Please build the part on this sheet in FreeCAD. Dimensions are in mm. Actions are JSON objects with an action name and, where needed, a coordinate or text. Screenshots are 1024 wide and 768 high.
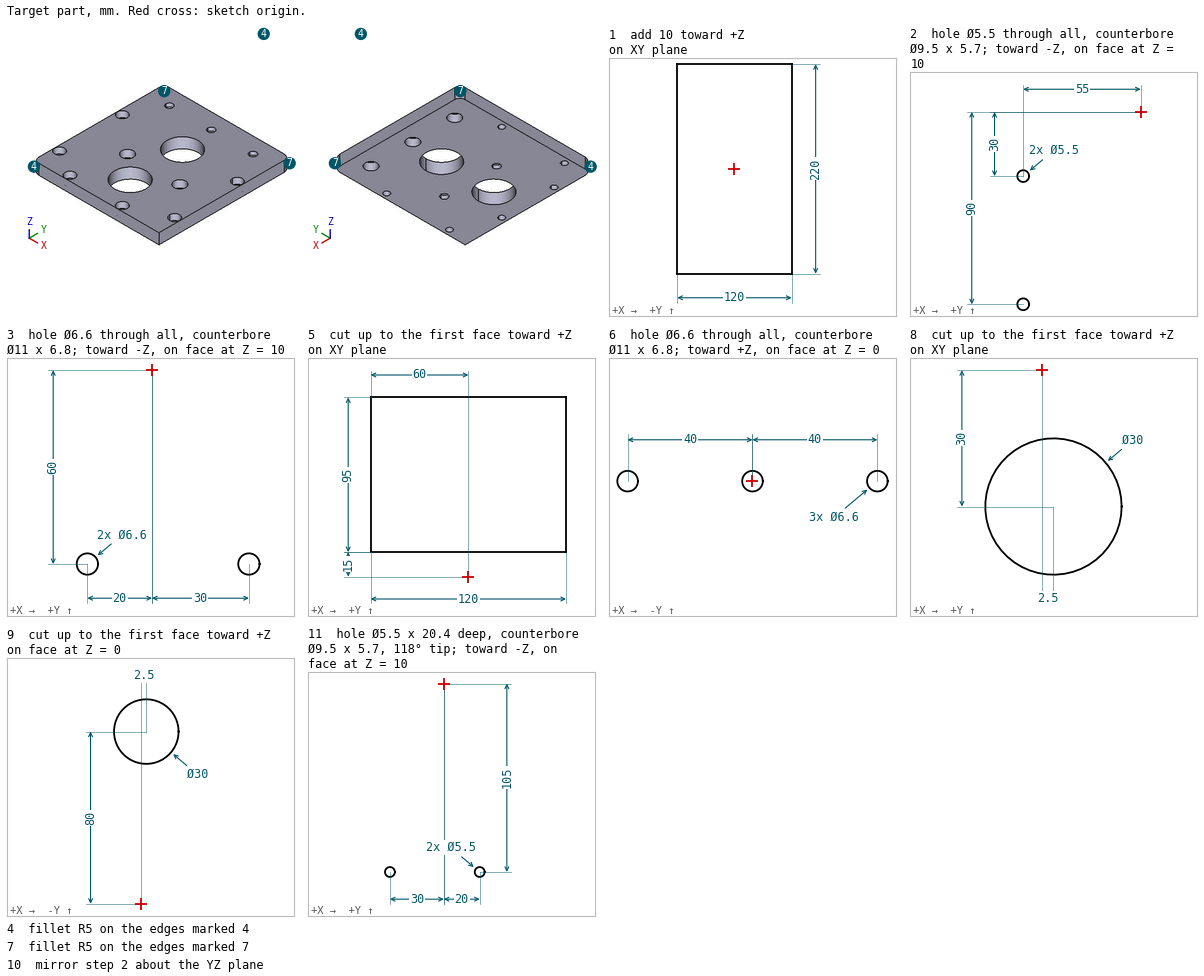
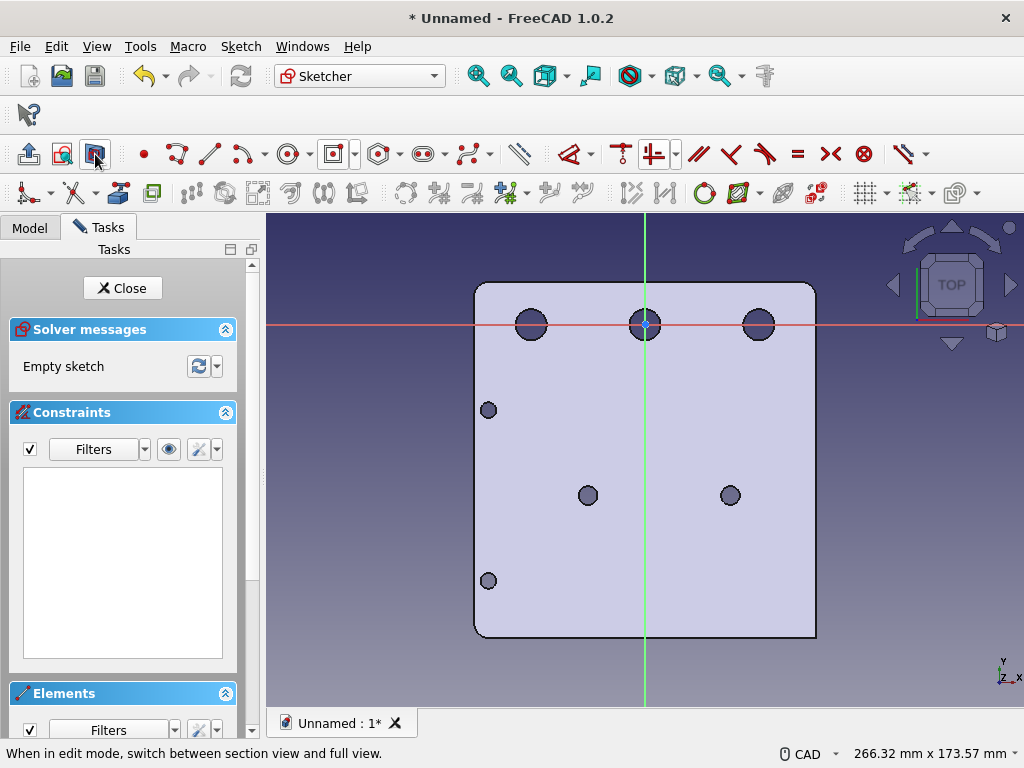
{"action": "scroll", "coordinate": [714, 331], "scroll_direction": "up", "scroll_amount": 4}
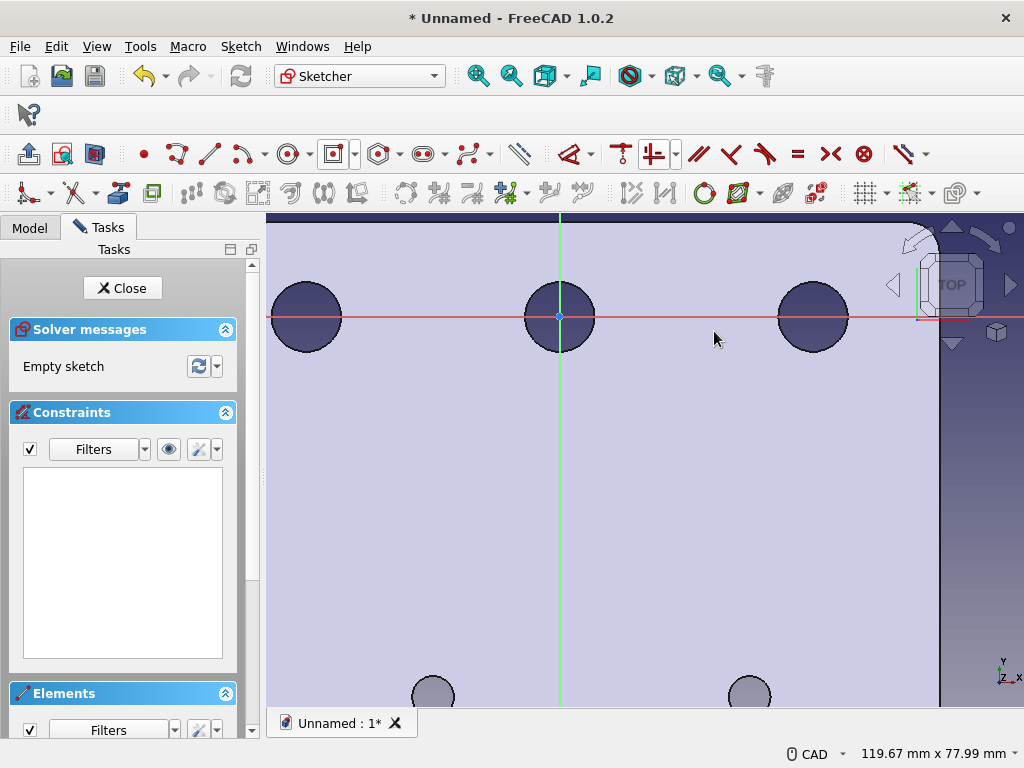
{"action": "left_click", "coordinate": [288, 154]}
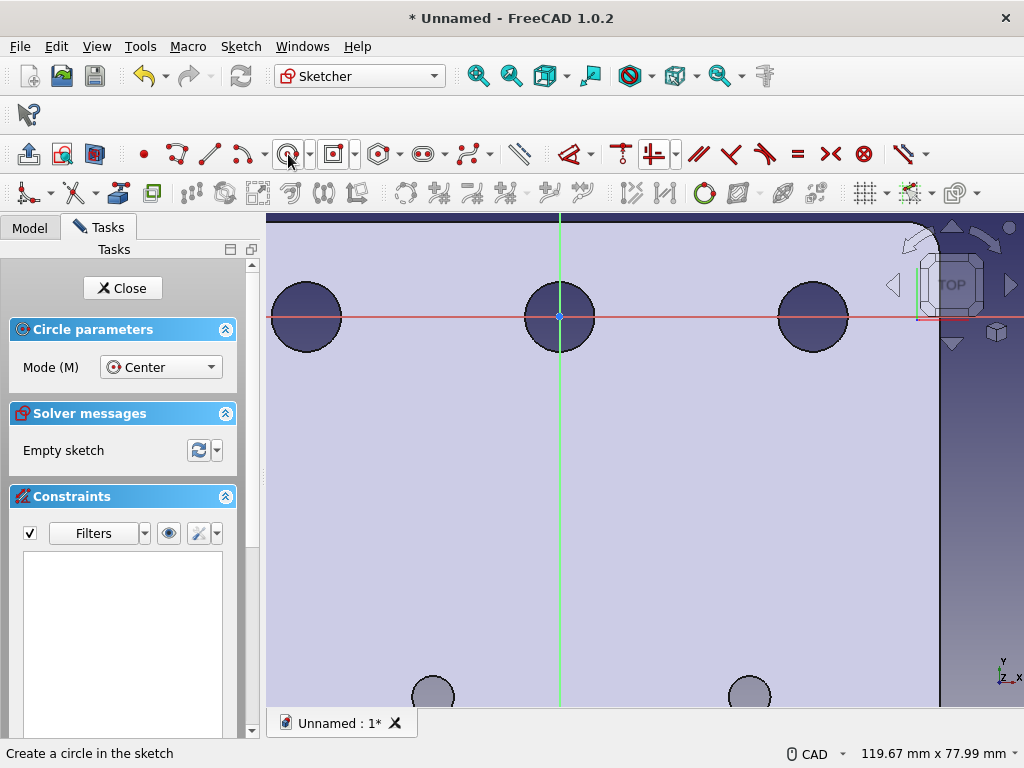
{"action": "left_click", "coordinate": [576, 507]}
{"action": "left_click", "coordinate": [643, 440]}
{"action": "key", "text": "Escape"}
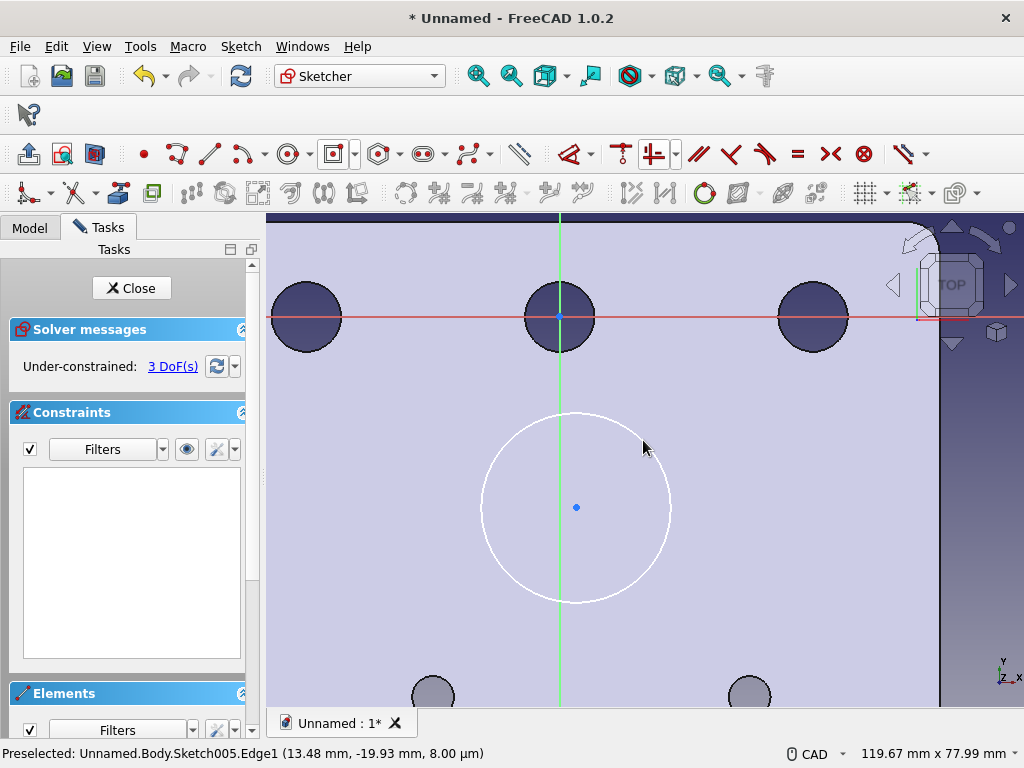
{"action": "left_click", "coordinate": [568, 154]}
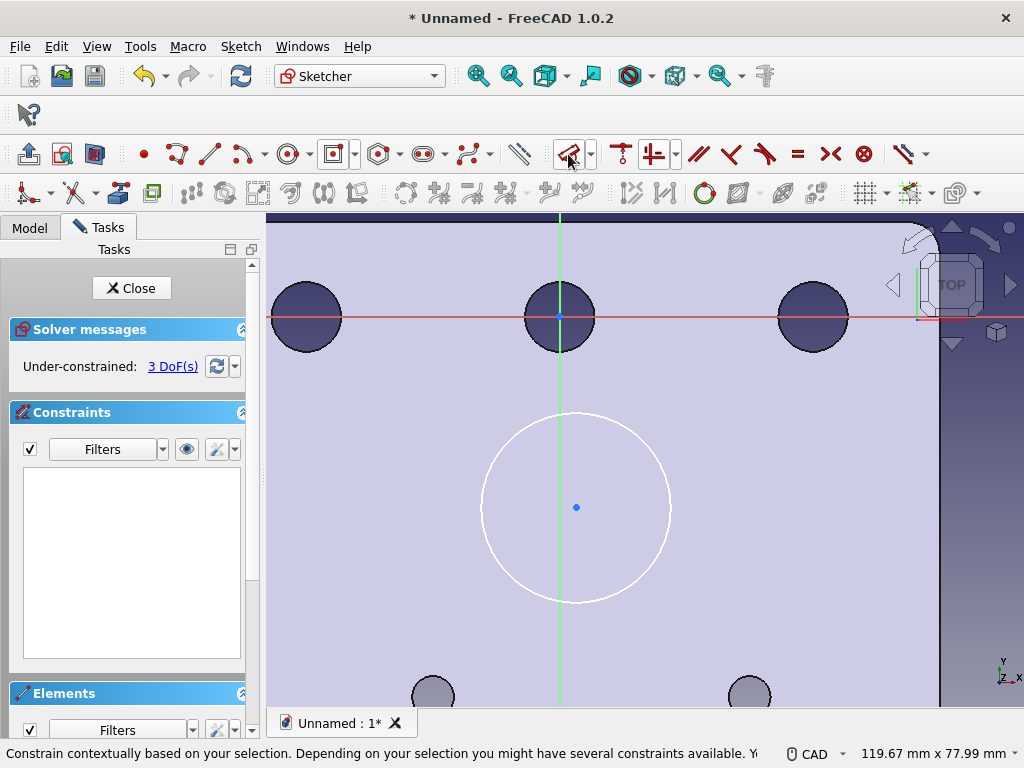
{"action": "left_click", "coordinate": [643, 441]}
{"action": "left_click", "coordinate": [666, 418]}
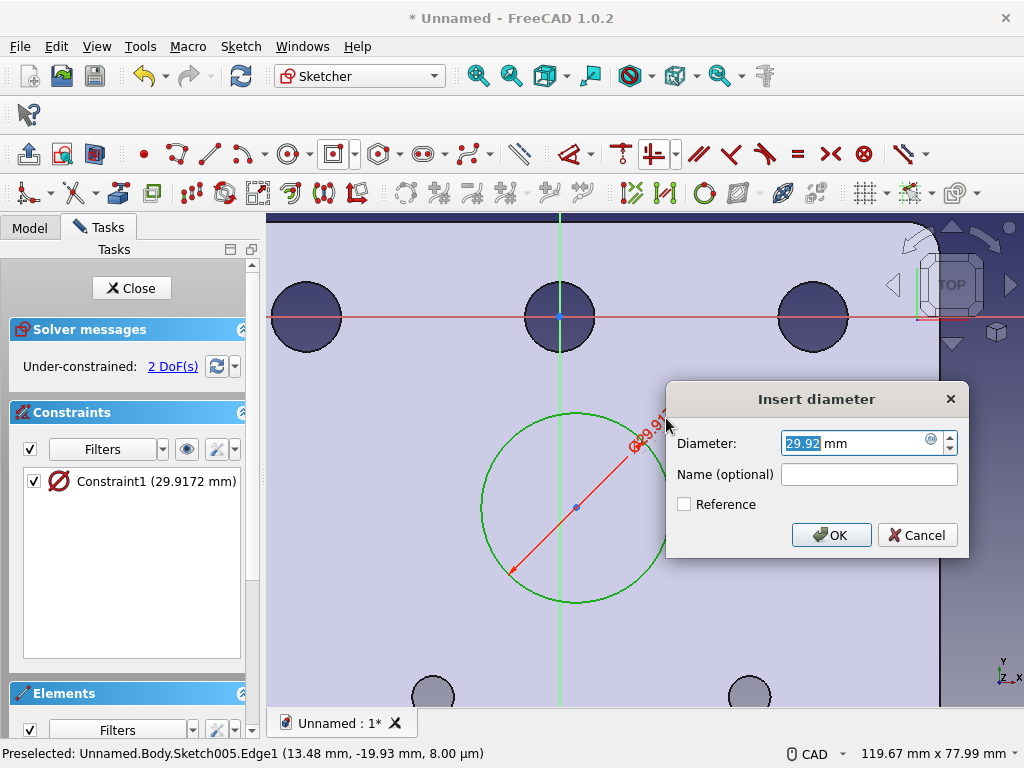
{"action": "type", "text": "30"}
{"action": "key", "text": "Return"}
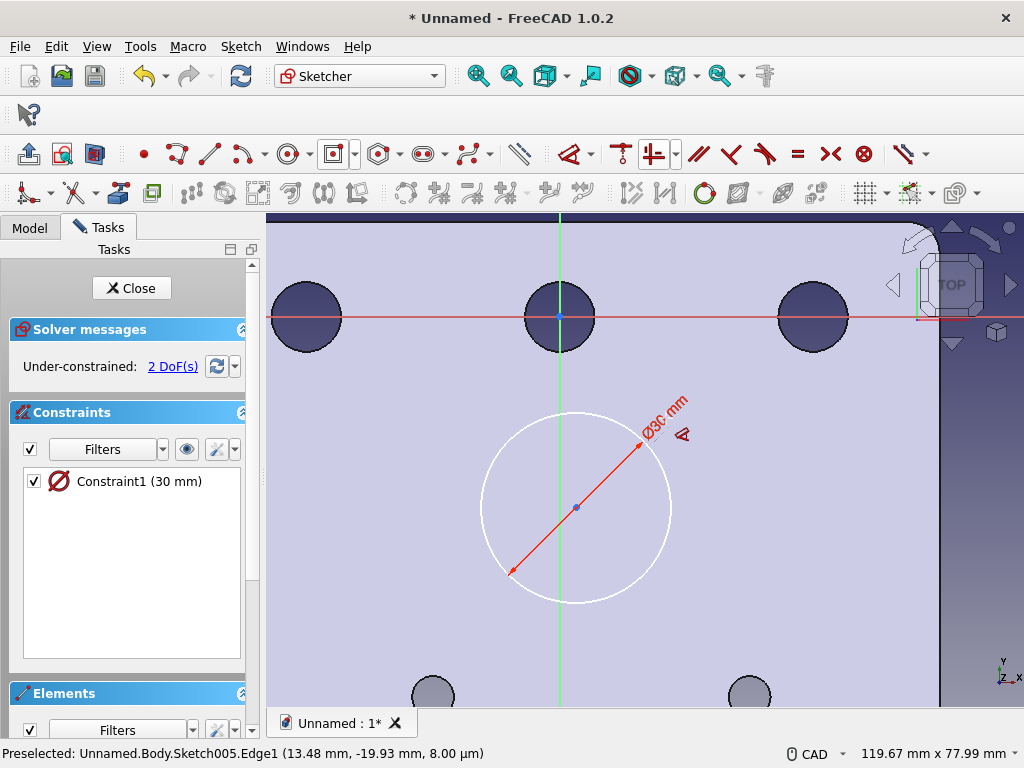
{"action": "left_click", "coordinate": [576, 508]}
{"action": "left_click", "coordinate": [526, 369]}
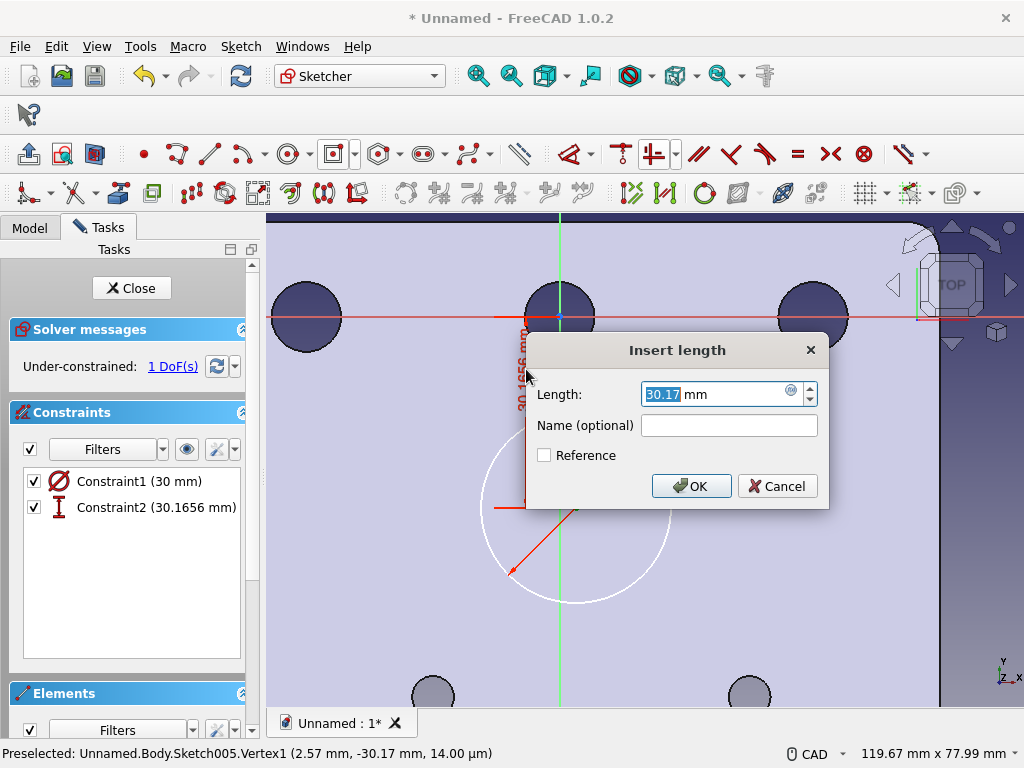
{"action": "type", "text": "30"}
{"action": "key", "text": "Return"}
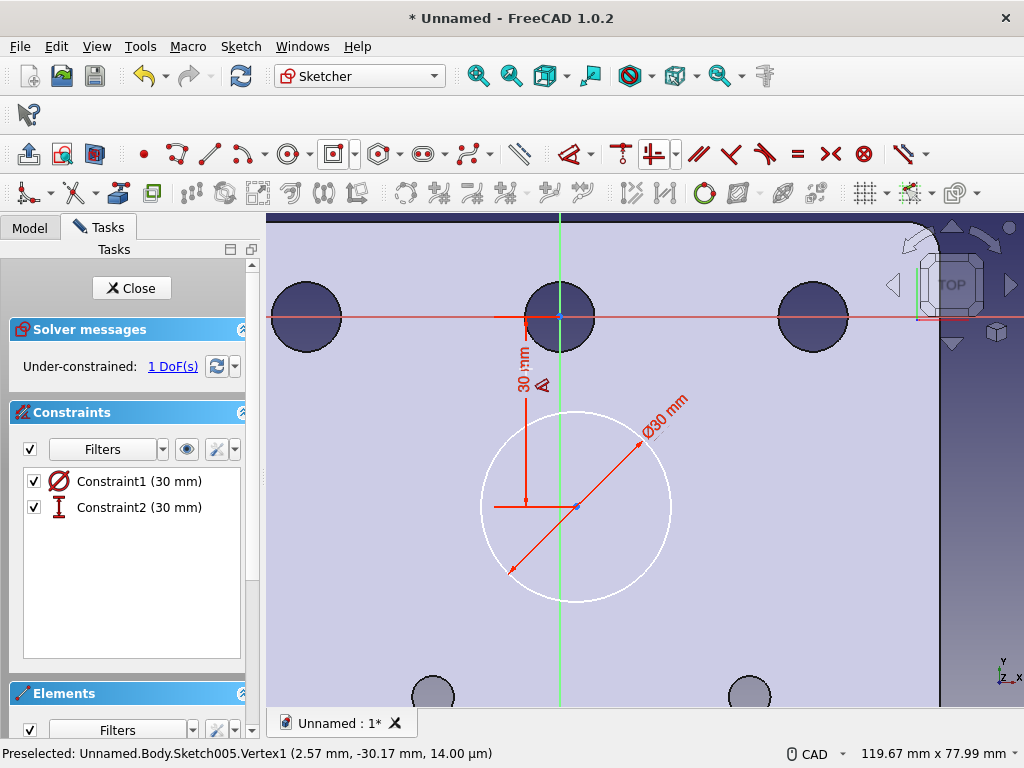
{"action": "scroll", "coordinate": [576, 507], "scroll_direction": "up", "scroll_amount": 5}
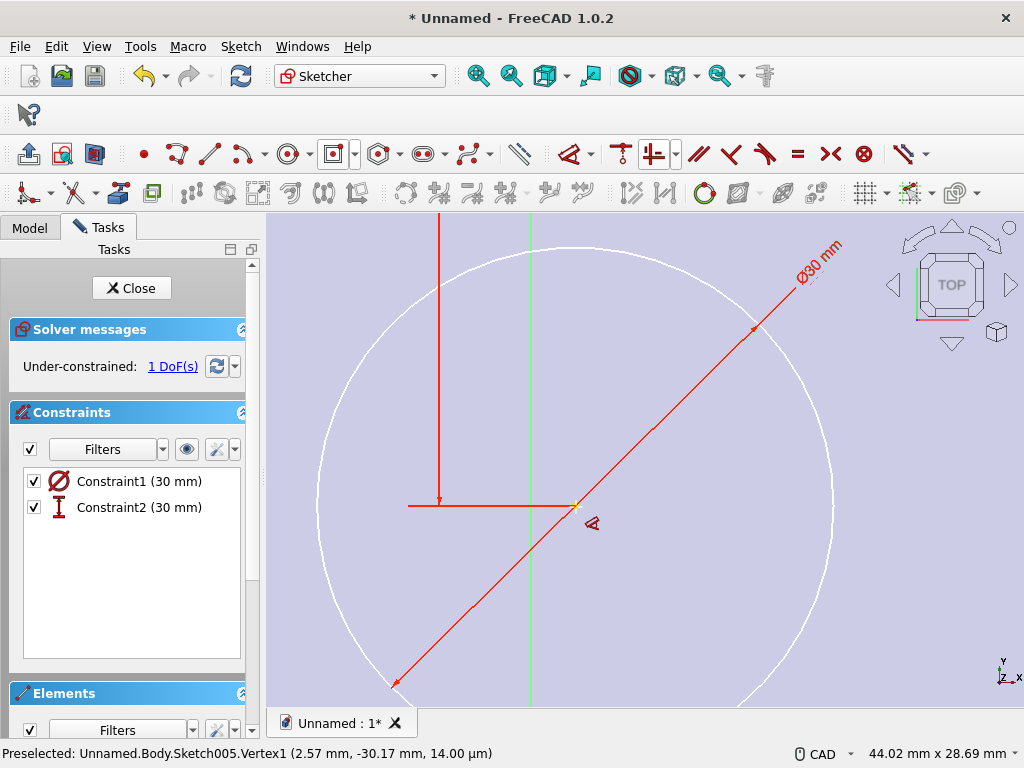
{"action": "left_click", "coordinate": [575, 506]}
{"action": "left_click", "coordinate": [553, 540]}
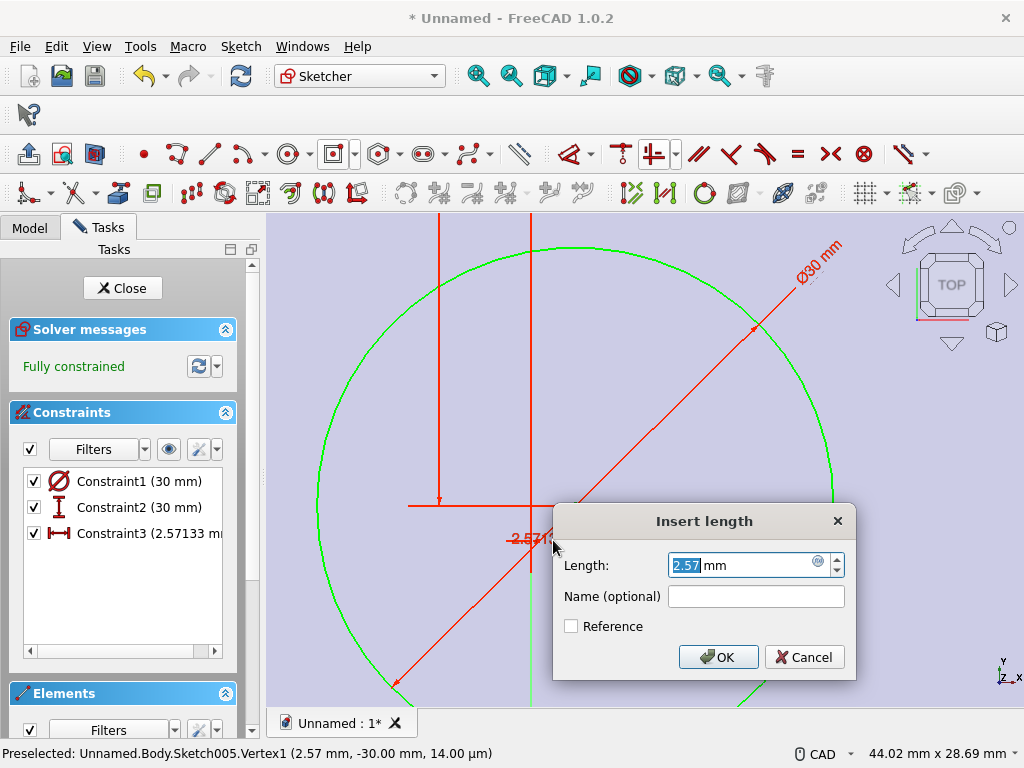
{"action": "type", "text": "2.5"}
{"action": "key", "text": "Return"}
{"action": "key", "text": "Escape"}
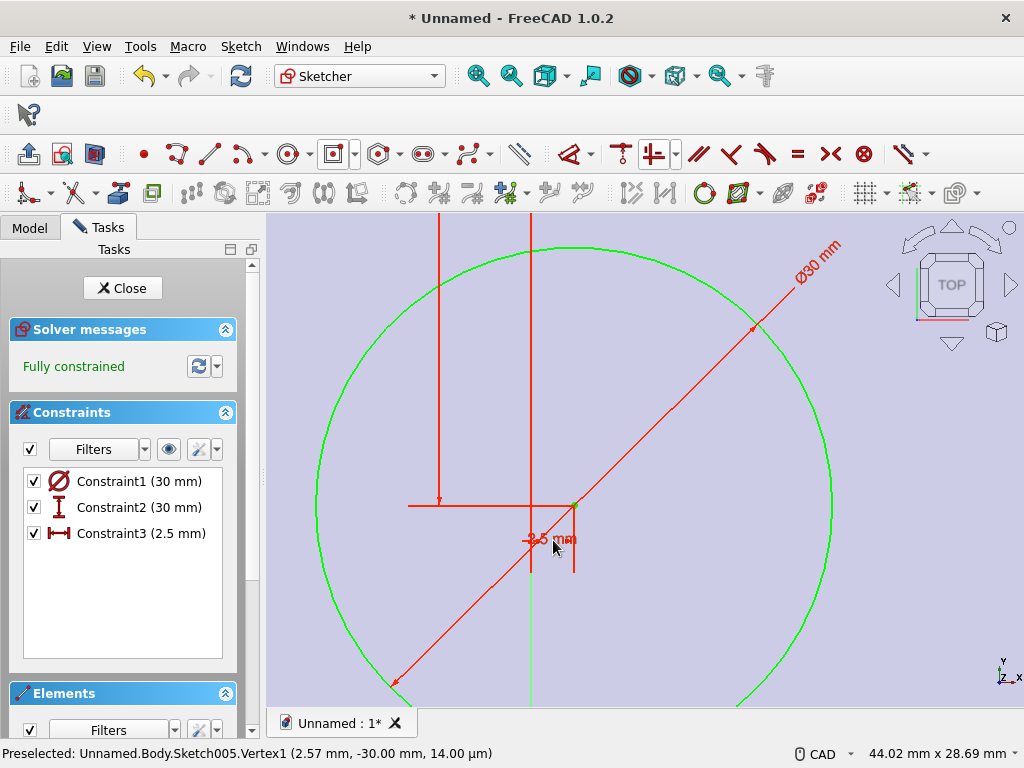
{"action": "left_click", "coordinate": [123, 288]}